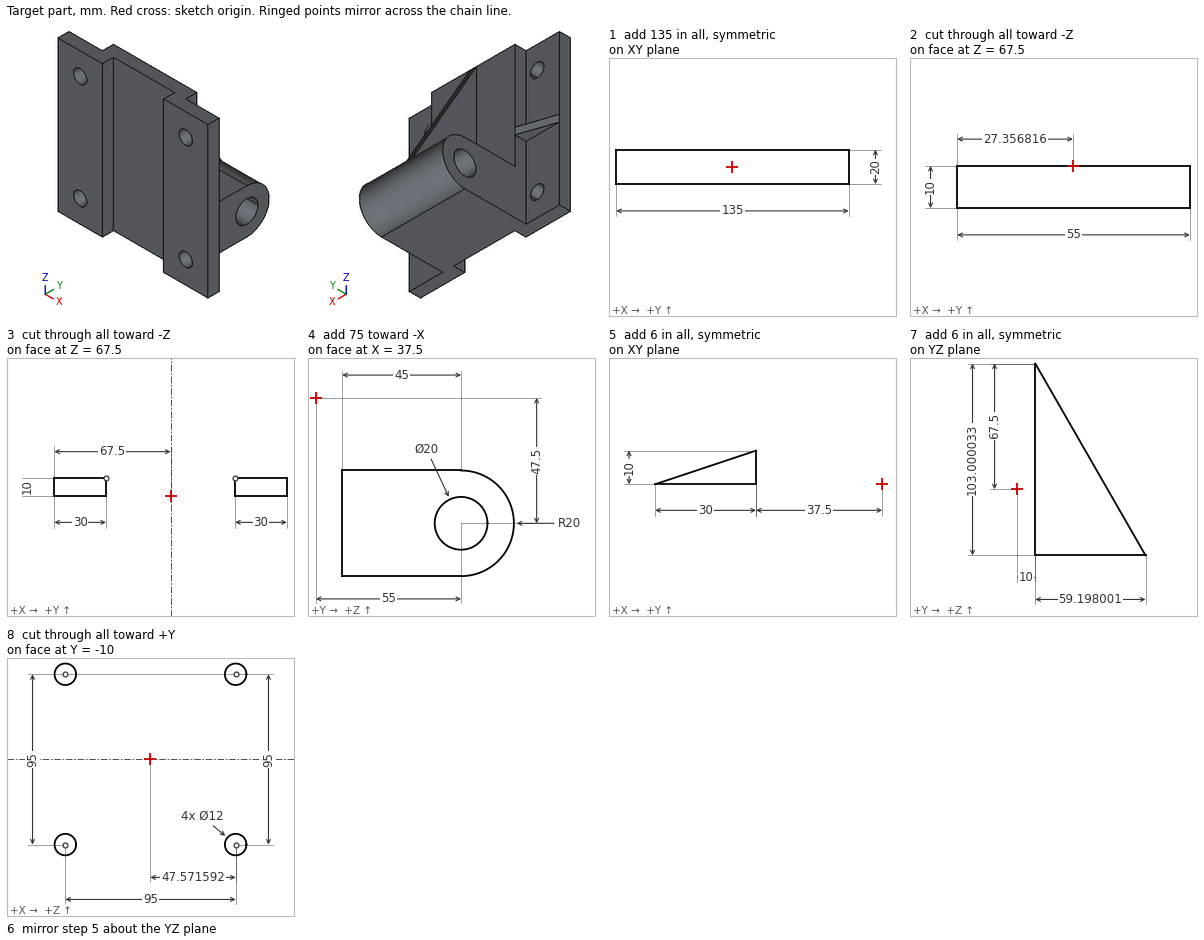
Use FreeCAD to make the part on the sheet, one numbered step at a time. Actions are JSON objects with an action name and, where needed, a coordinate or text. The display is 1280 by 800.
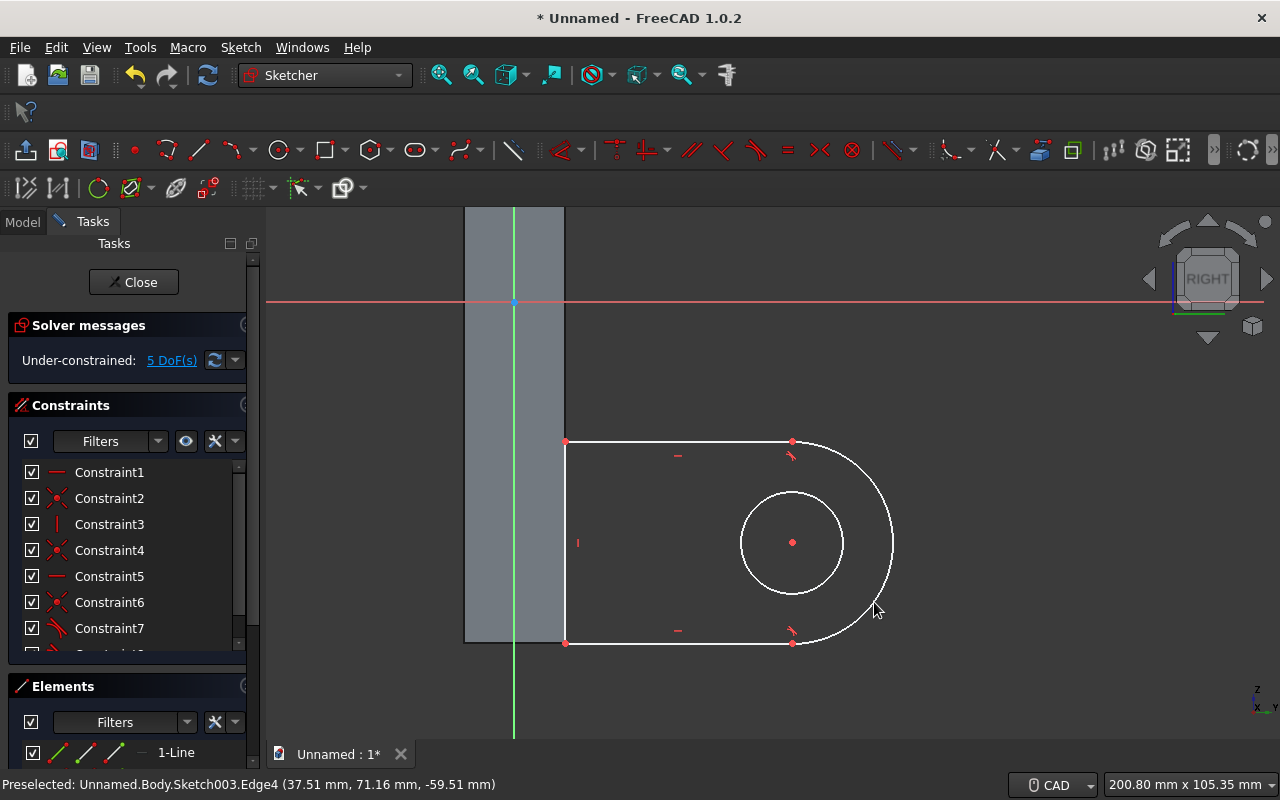
{"action": "left_click", "coordinate": [560, 150]}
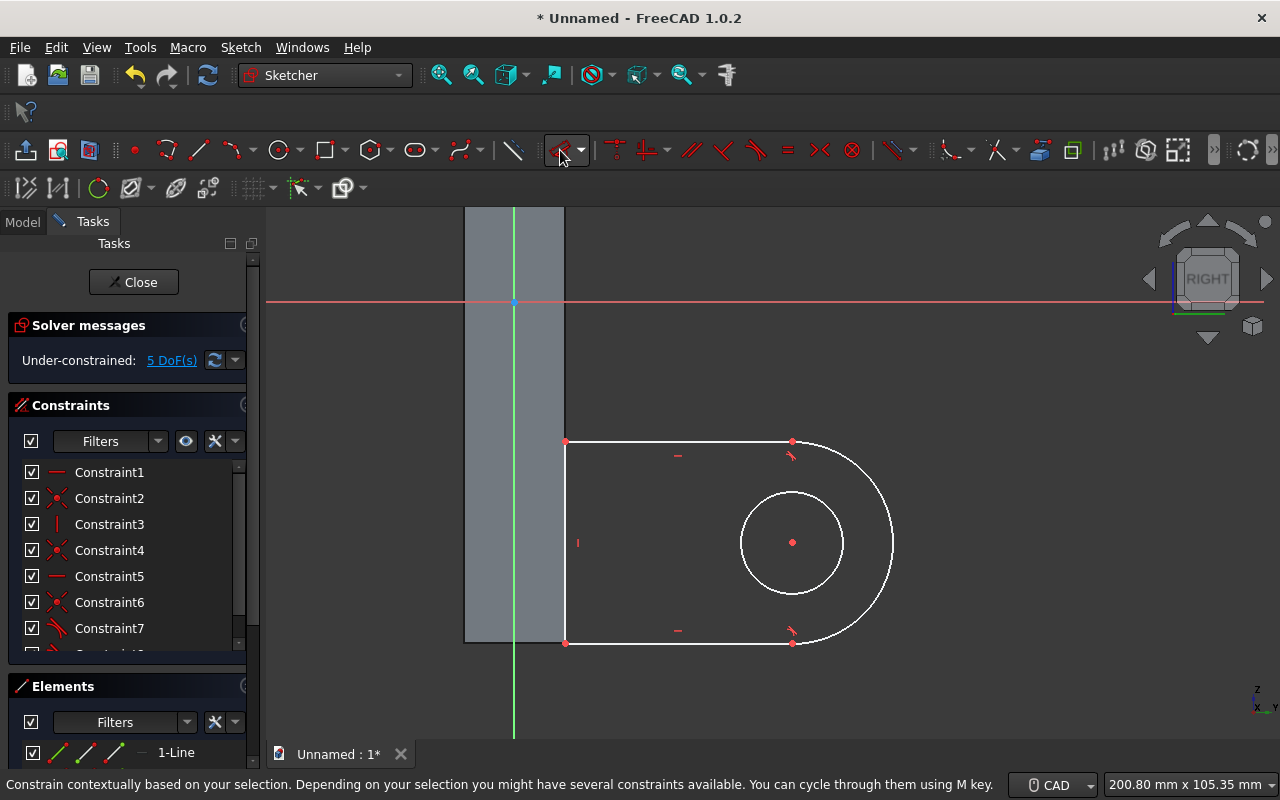
{"action": "left_click", "coordinate": [874, 602]}
{"action": "left_click", "coordinate": [900, 621]}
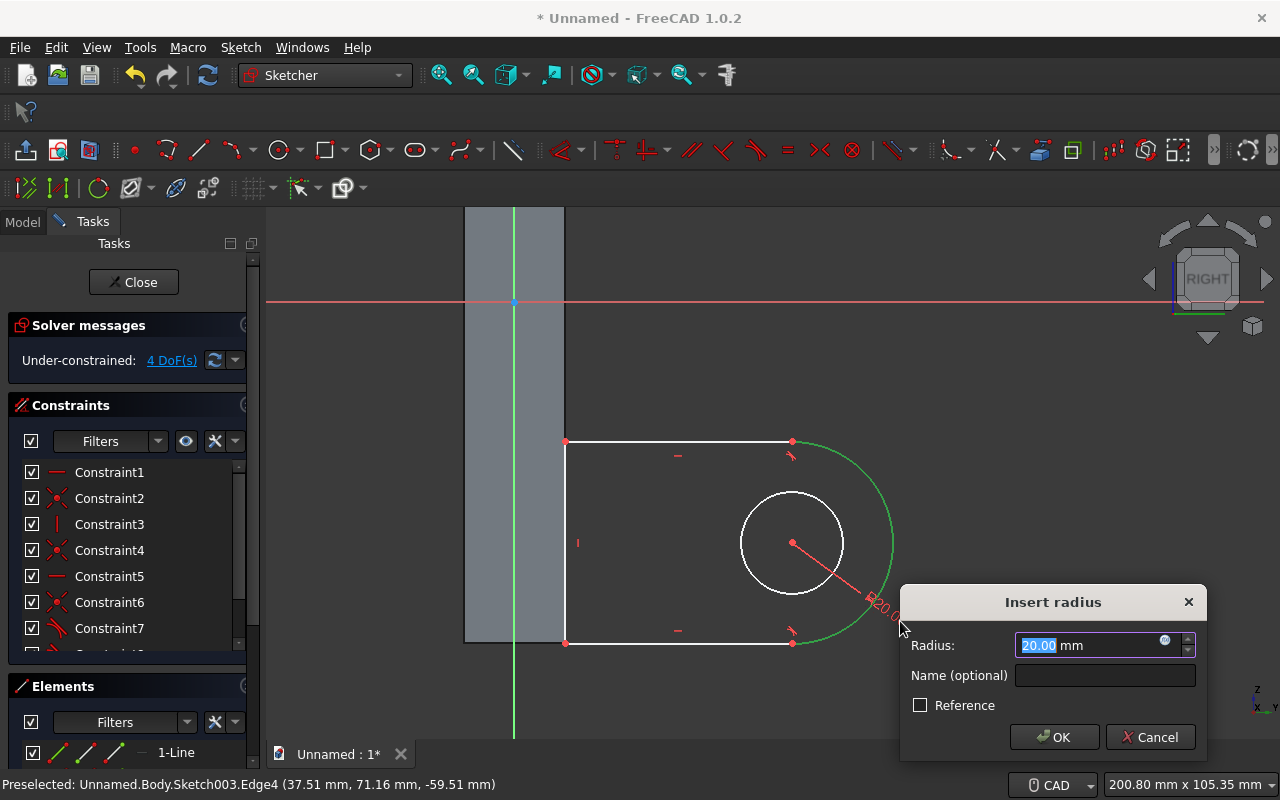
{"action": "type", "text": "20"}
{"action": "key", "text": "Return"}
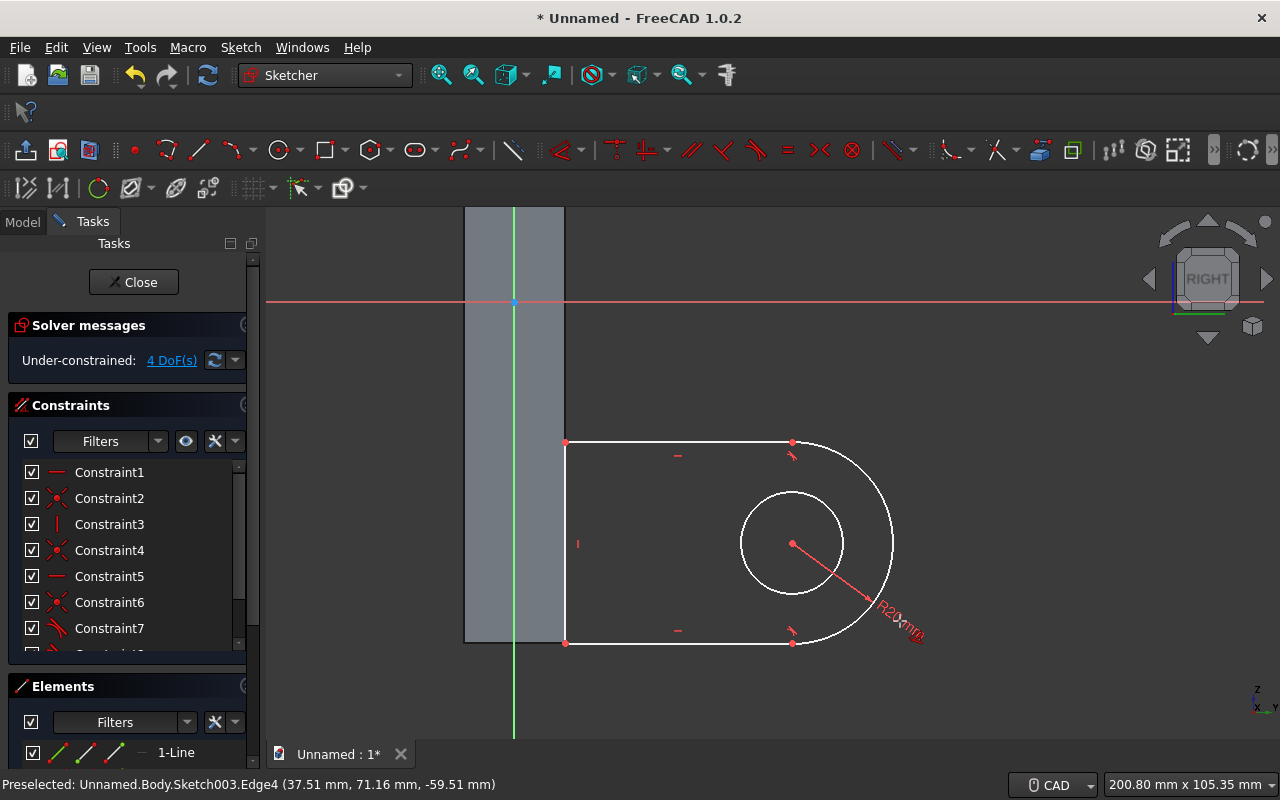
{"action": "left_click", "coordinate": [828, 507]}
{"action": "left_click", "coordinate": [851, 484]}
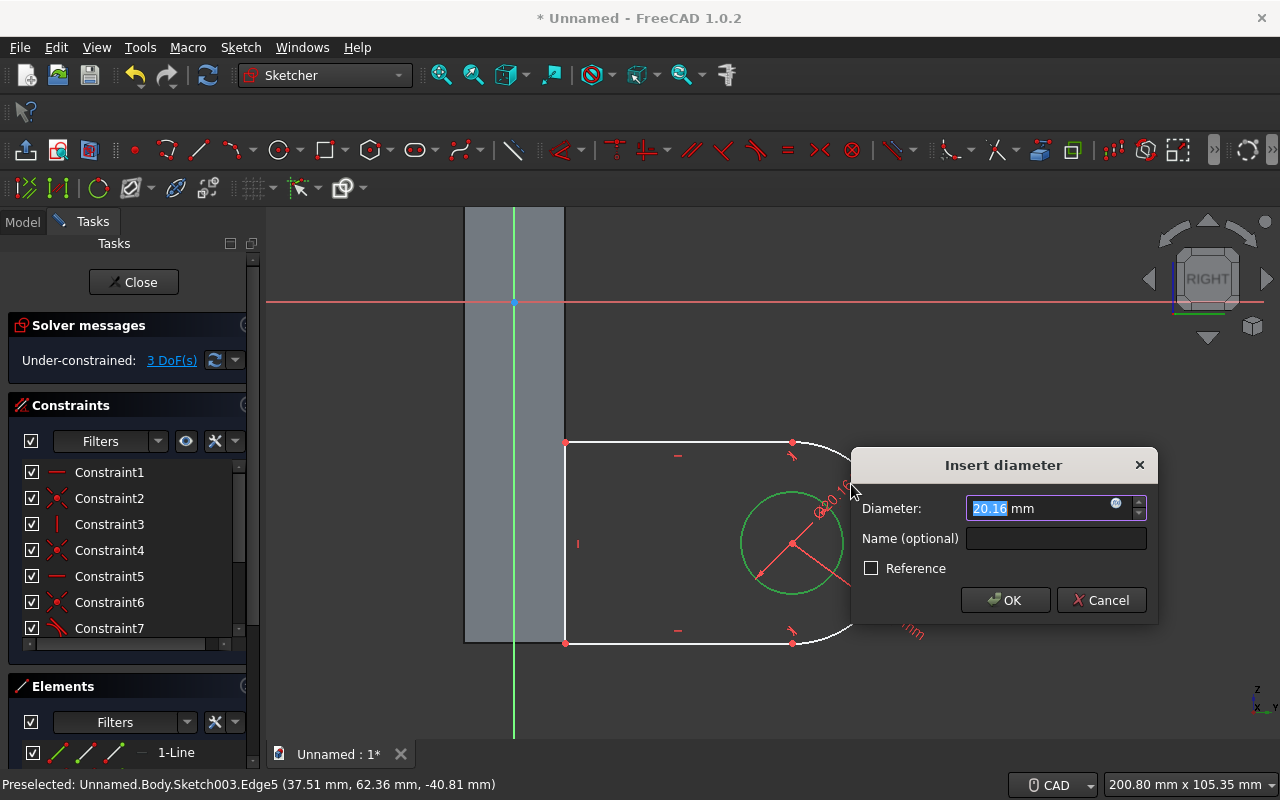
{"action": "type", "text": "20"}
{"action": "key", "text": "Return"}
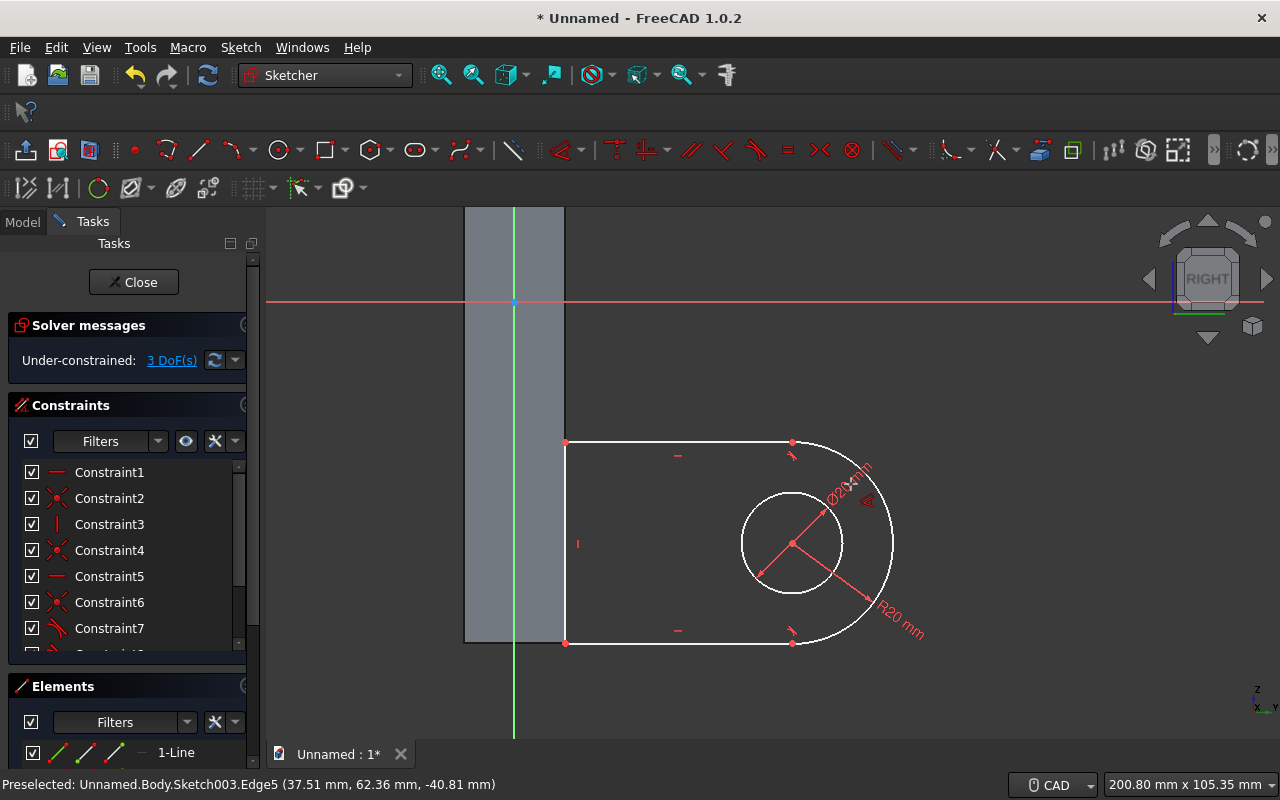
{"action": "left_click", "coordinate": [724, 442]}
{"action": "left_click", "coordinate": [678, 408]}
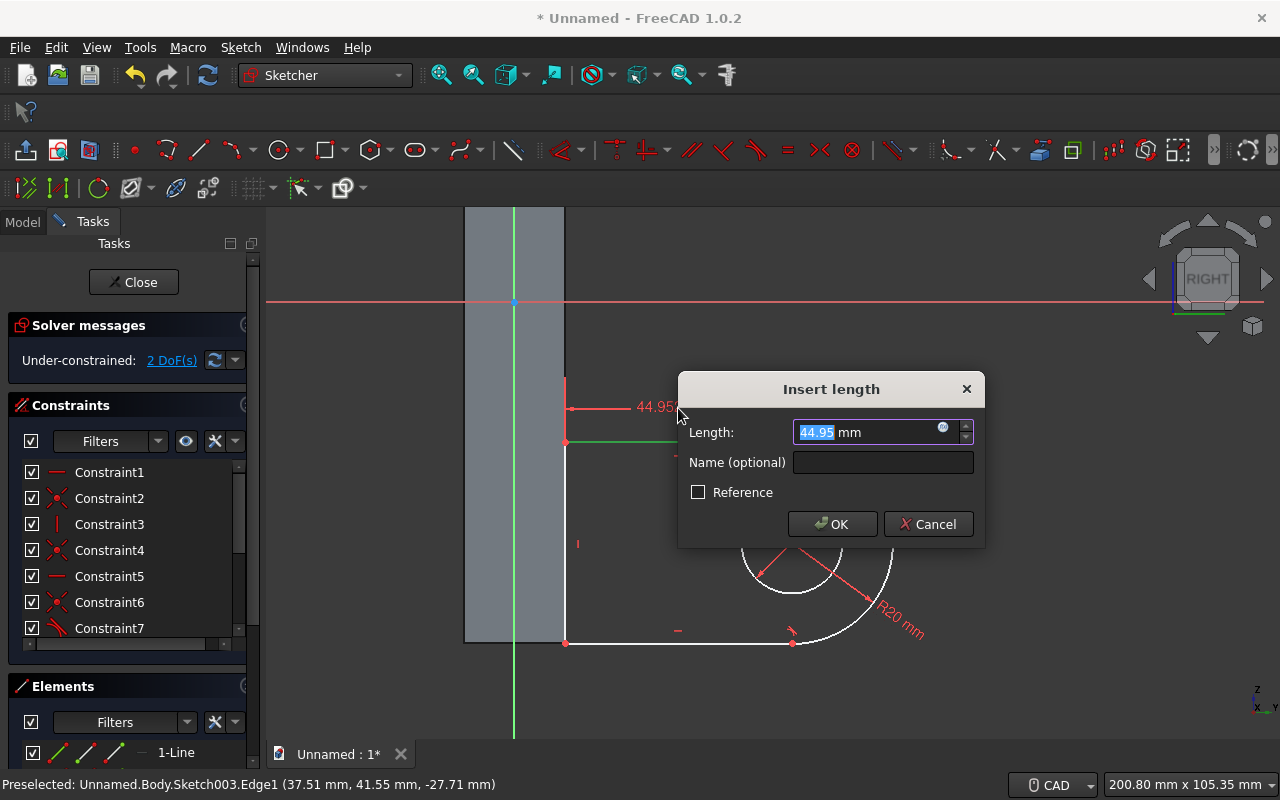
{"action": "type", "text": "45"}
{"action": "key", "text": "Return"}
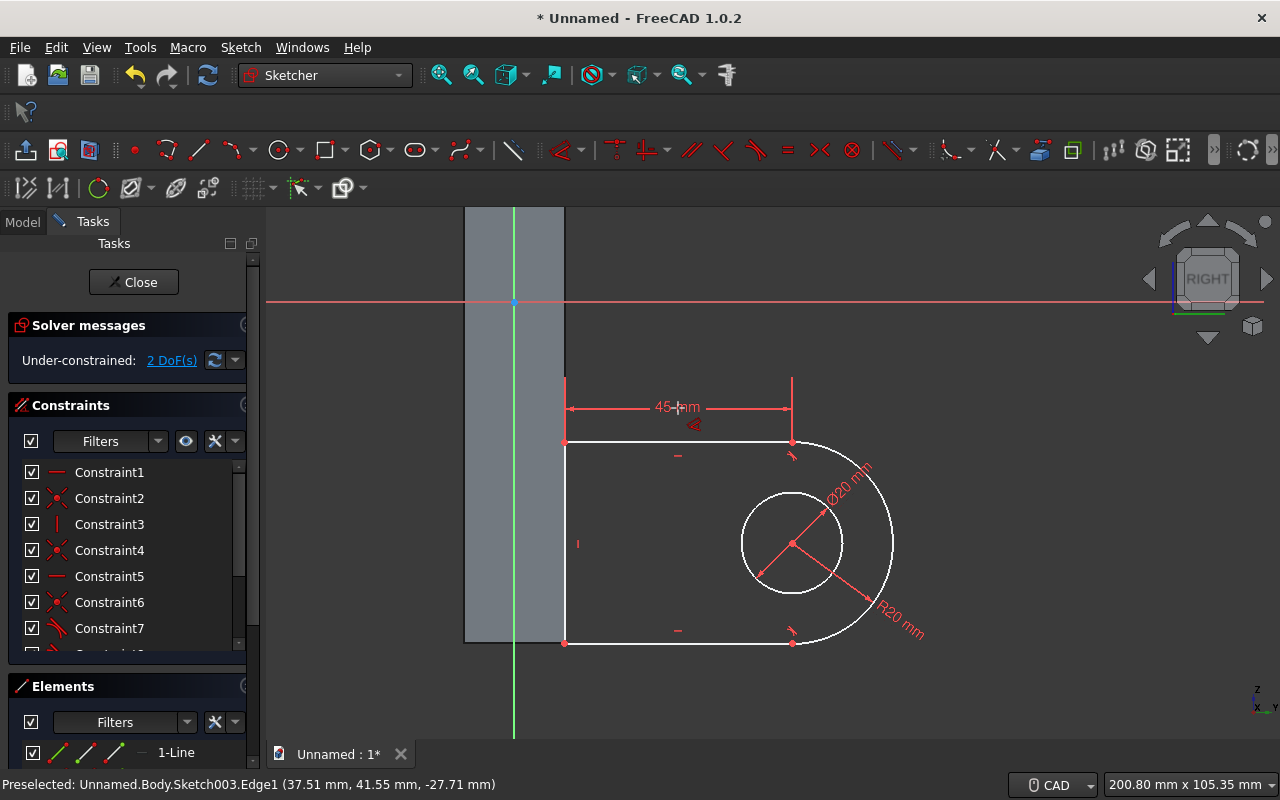
{"action": "left_click", "coordinate": [792, 543]}
{"action": "left_click", "coordinate": [653, 268]}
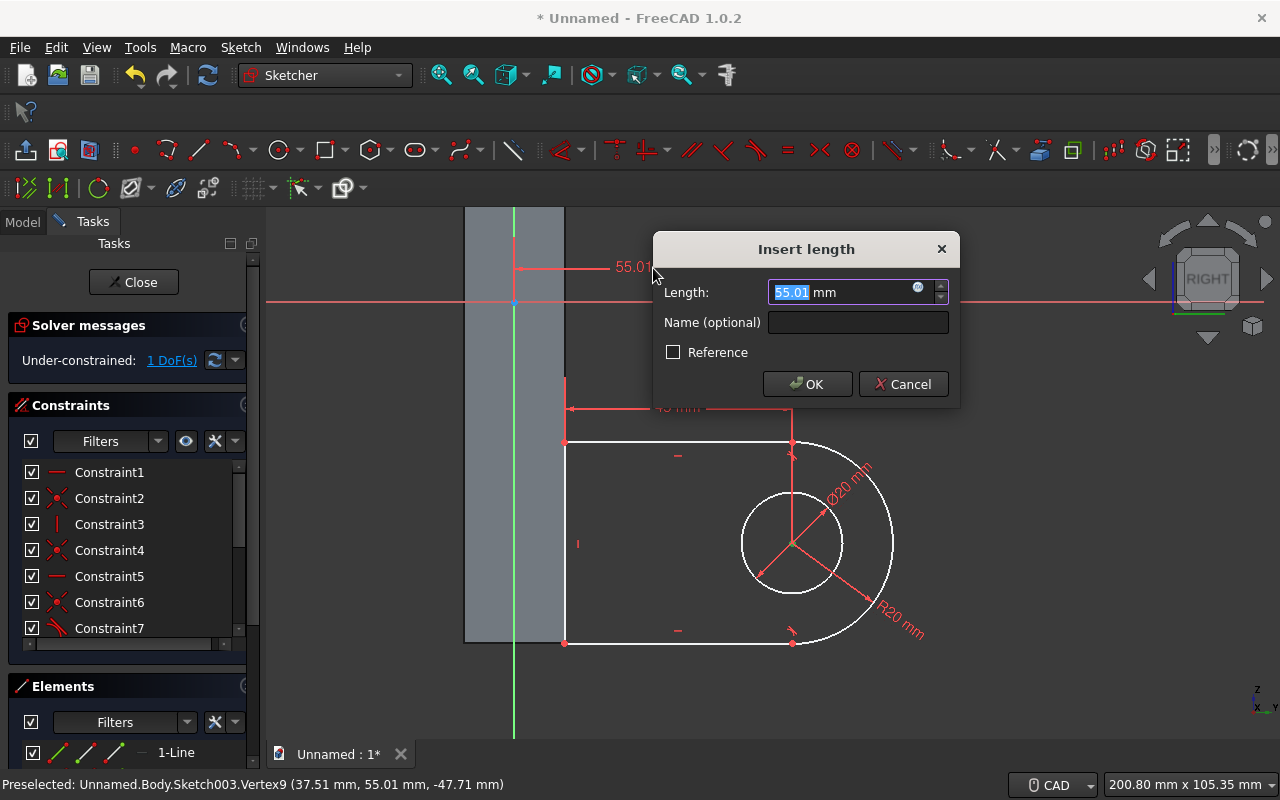
{"action": "type", "text": "55"}
{"action": "key", "text": "Return"}